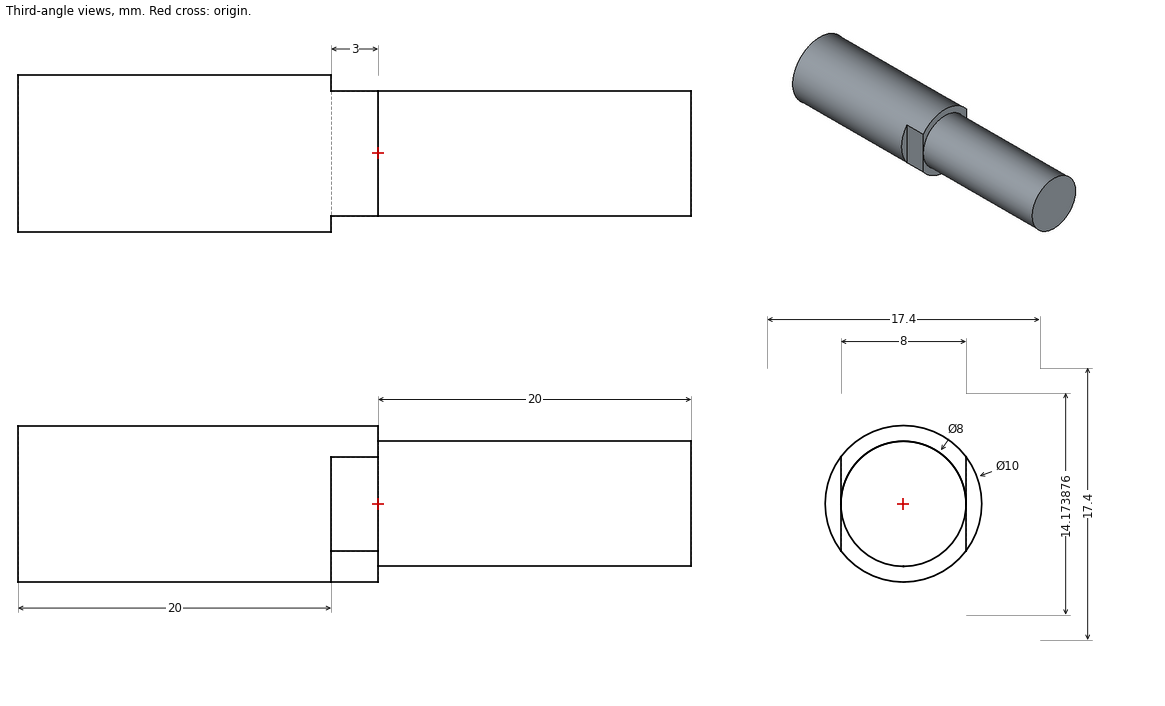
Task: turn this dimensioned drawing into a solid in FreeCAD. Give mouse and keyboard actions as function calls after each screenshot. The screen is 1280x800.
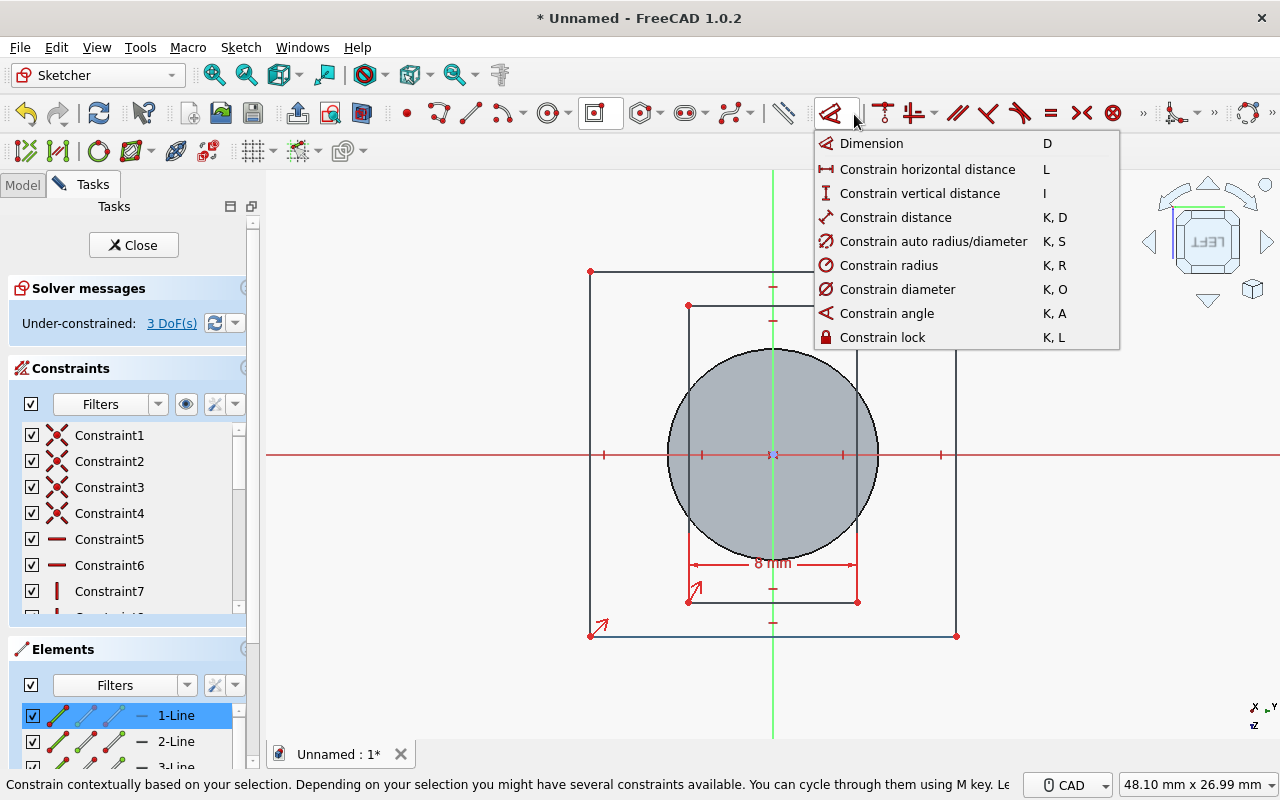
click(967, 169)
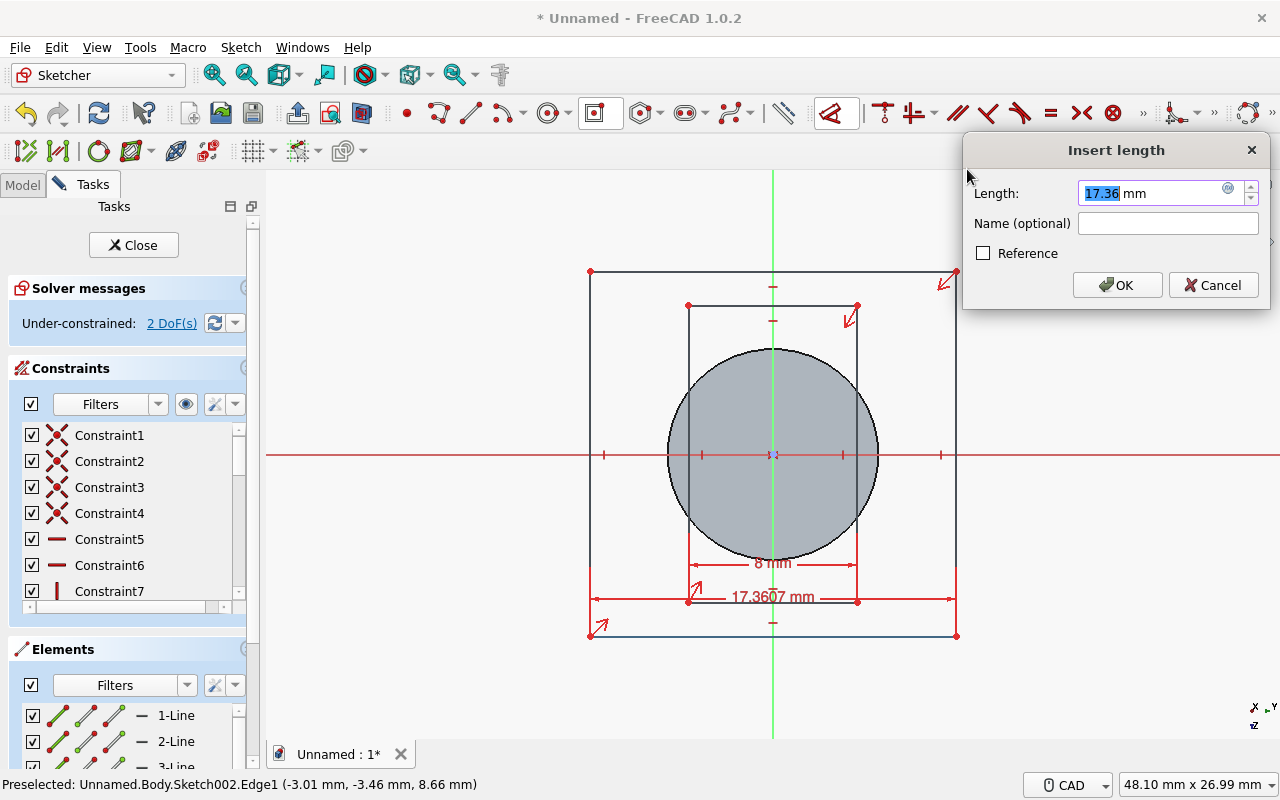
text(17.4)
key(Return)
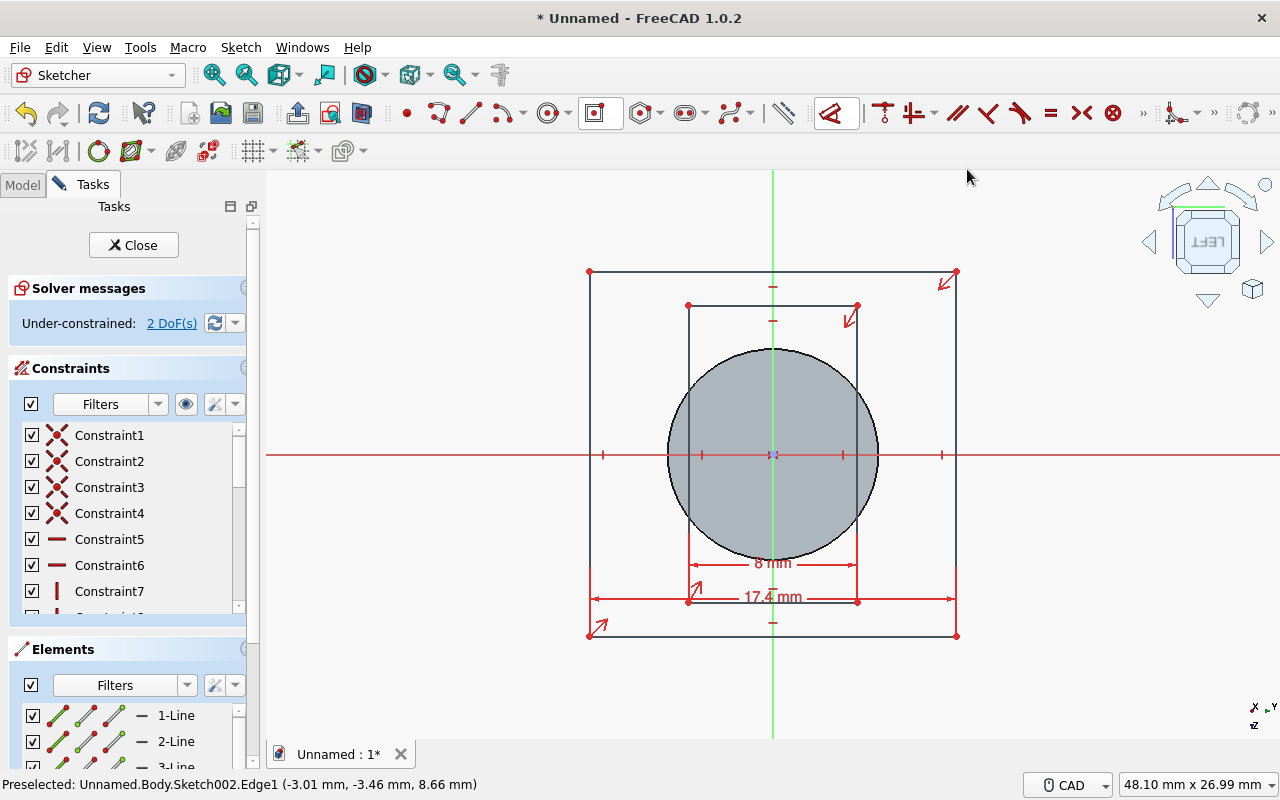
click(956, 527)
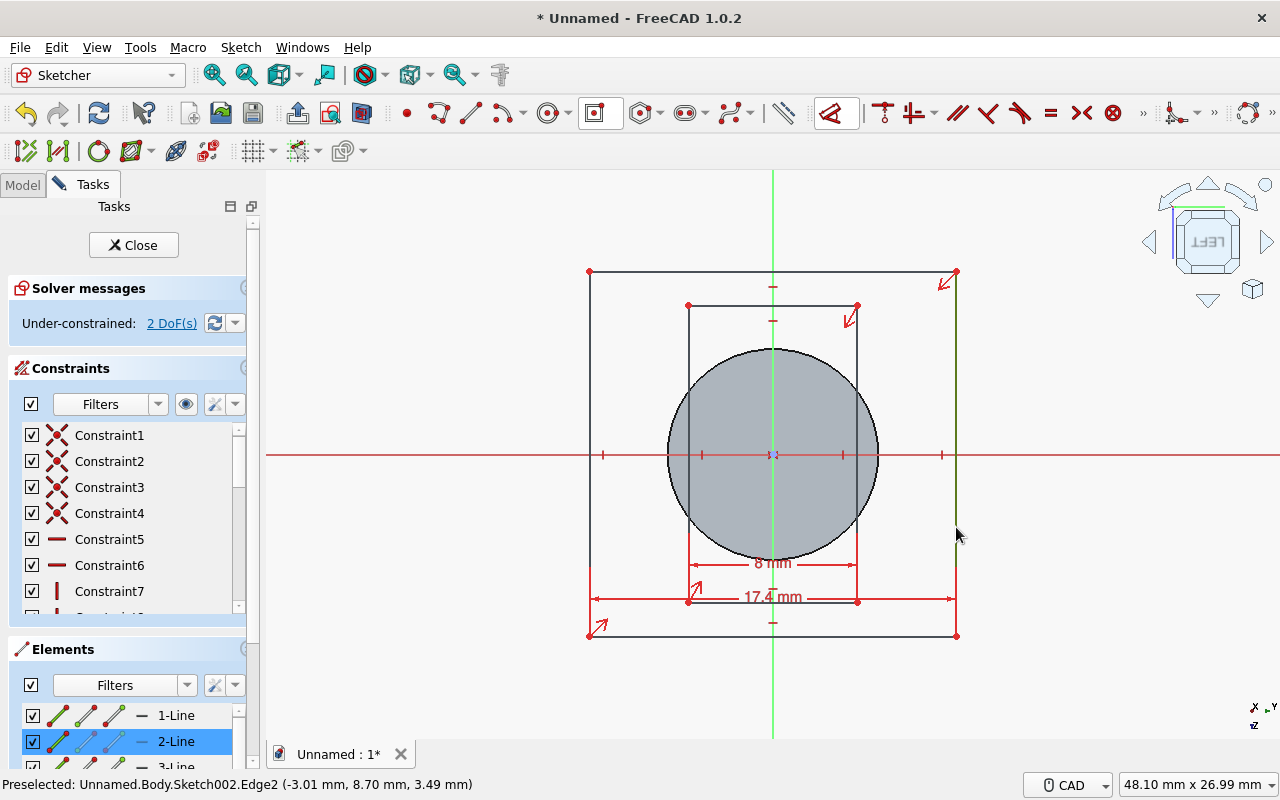
key(i)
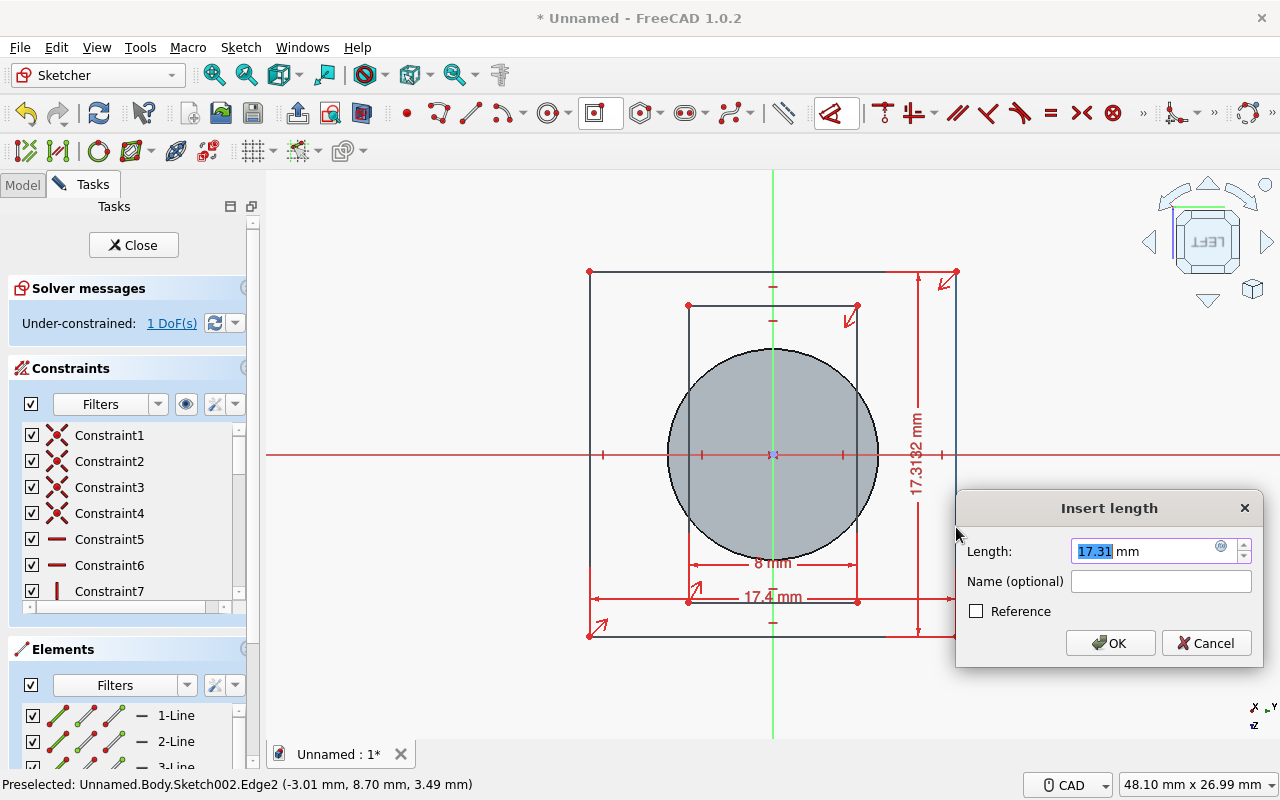
text(17.4)
key(Return)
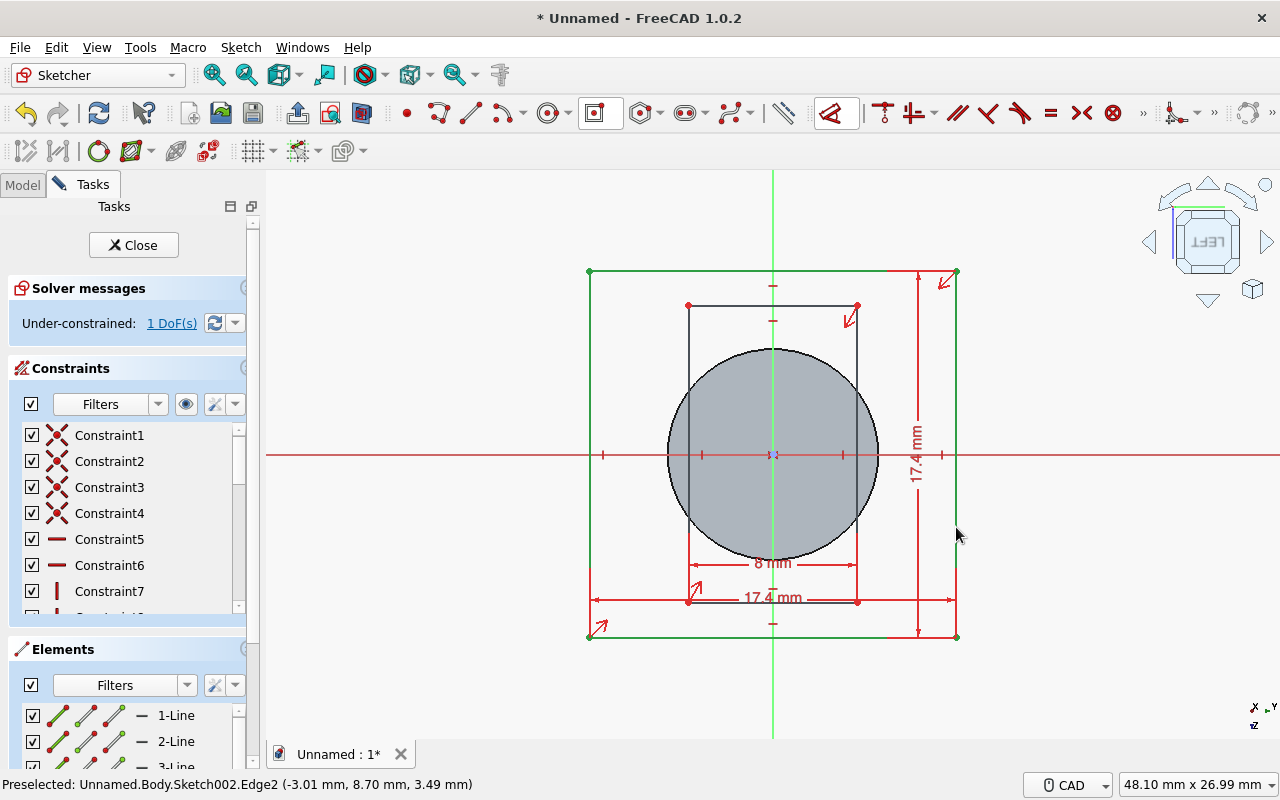
click(857, 514)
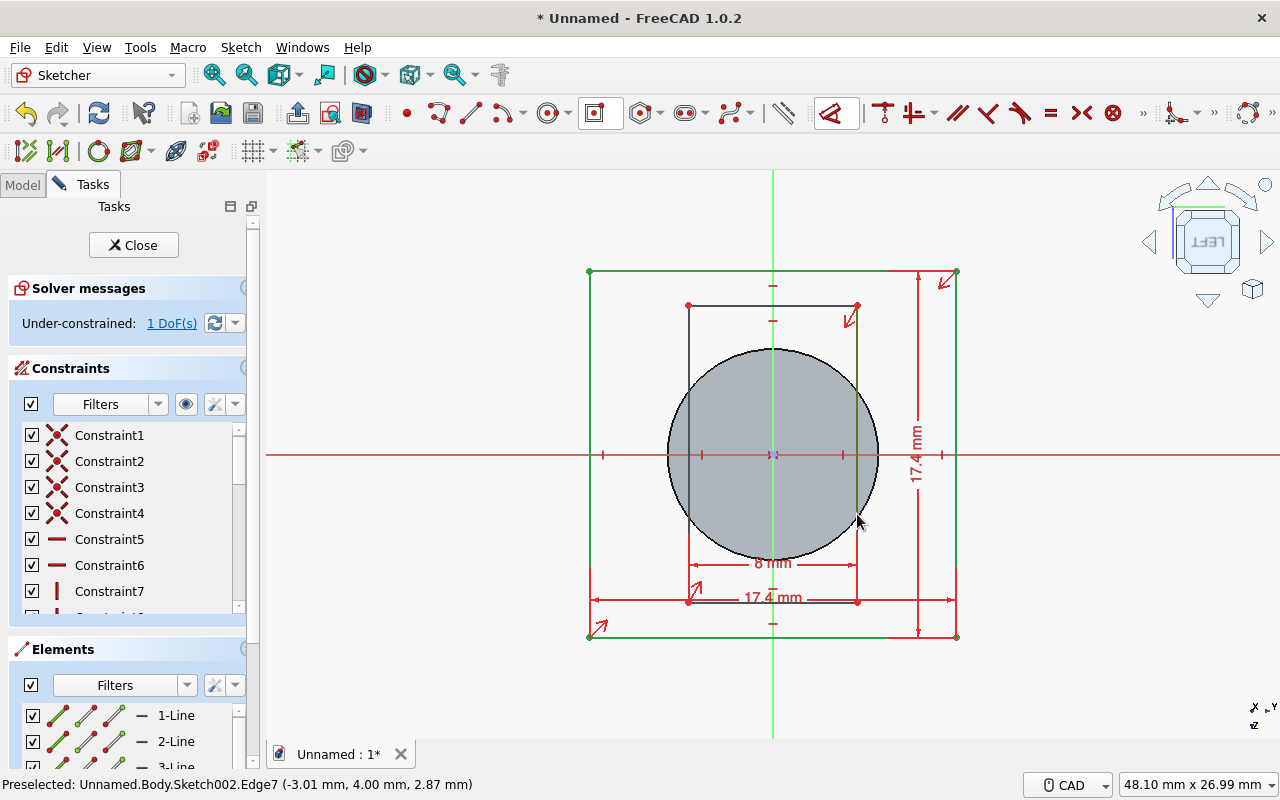
key(i)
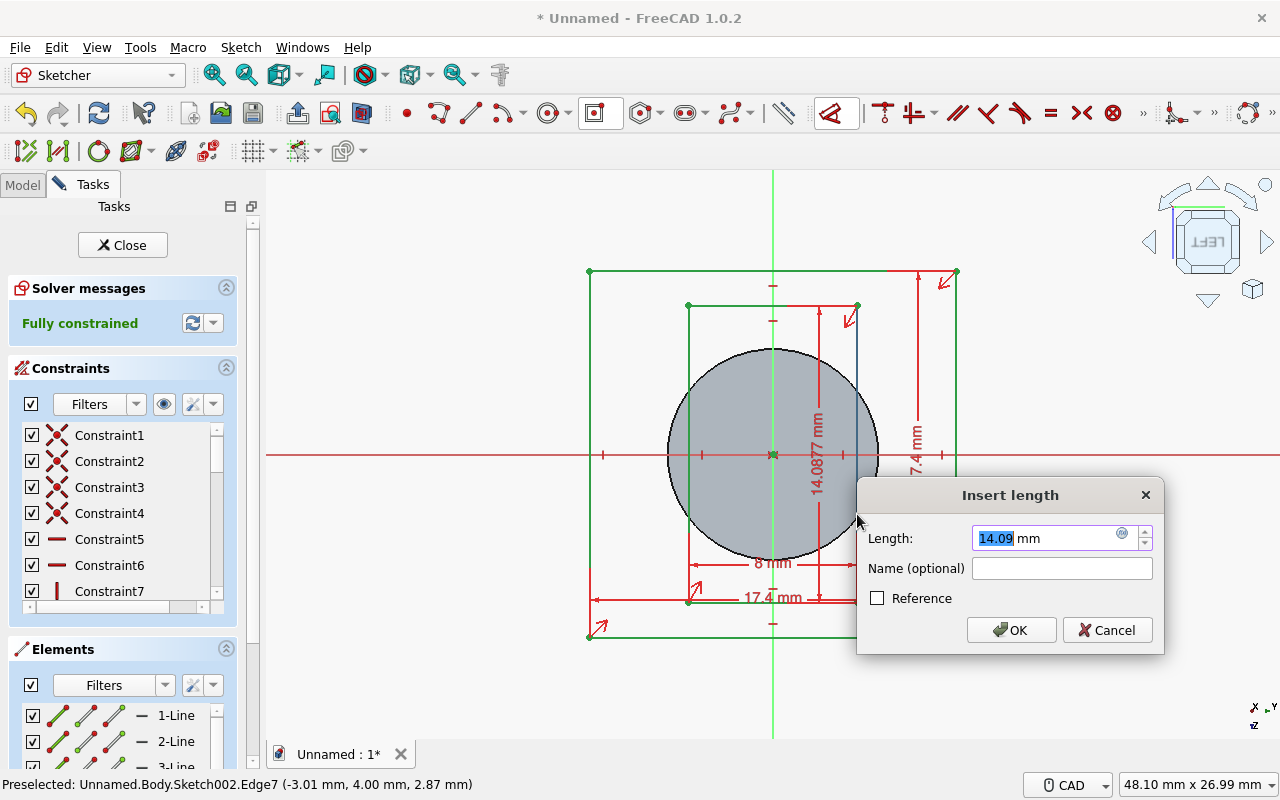
text(14.173876)
key(Return)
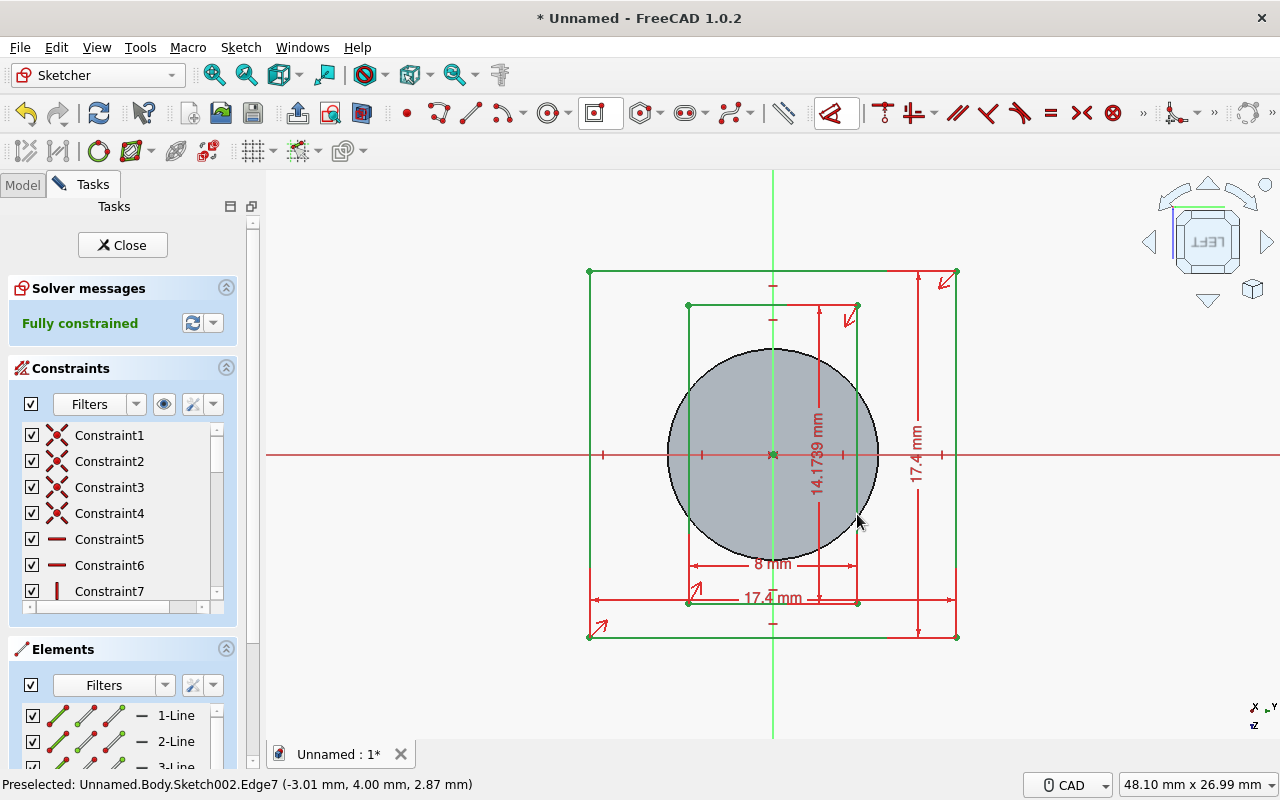
click(123, 245)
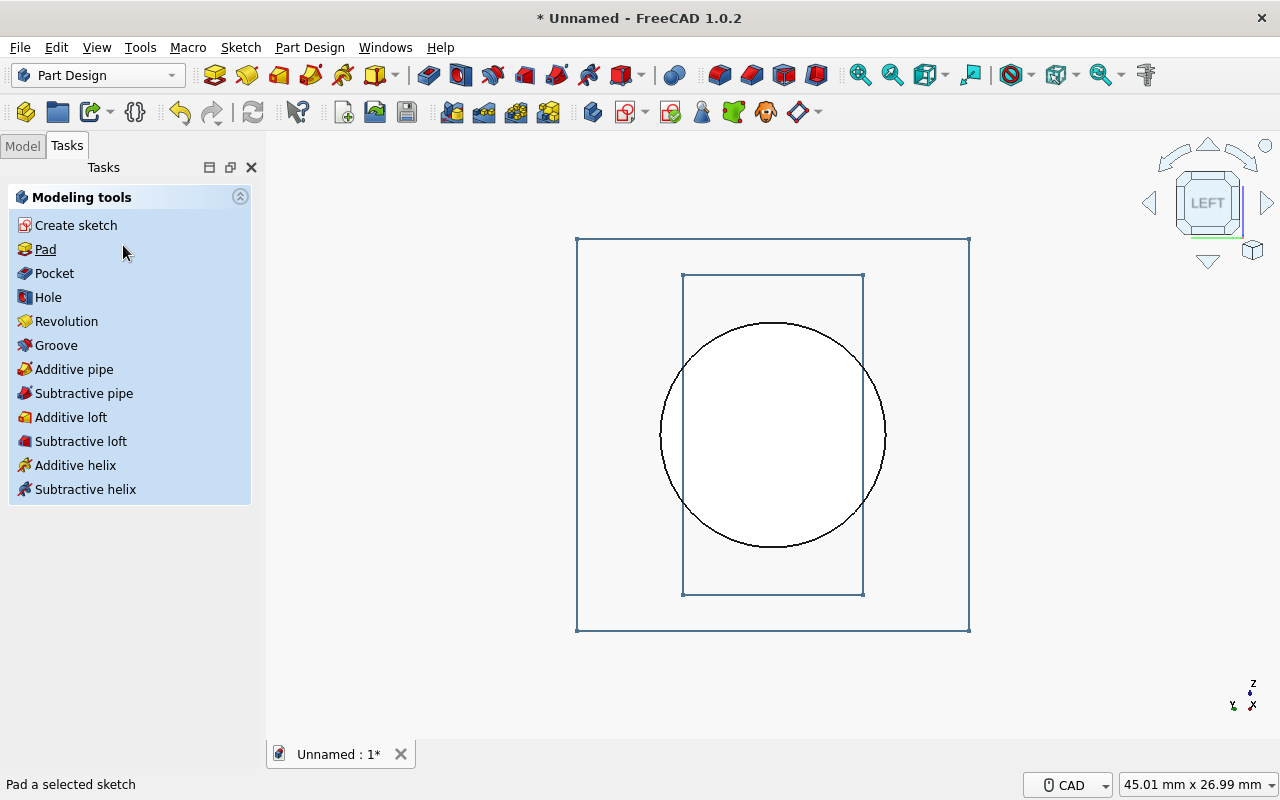
click(430, 76)